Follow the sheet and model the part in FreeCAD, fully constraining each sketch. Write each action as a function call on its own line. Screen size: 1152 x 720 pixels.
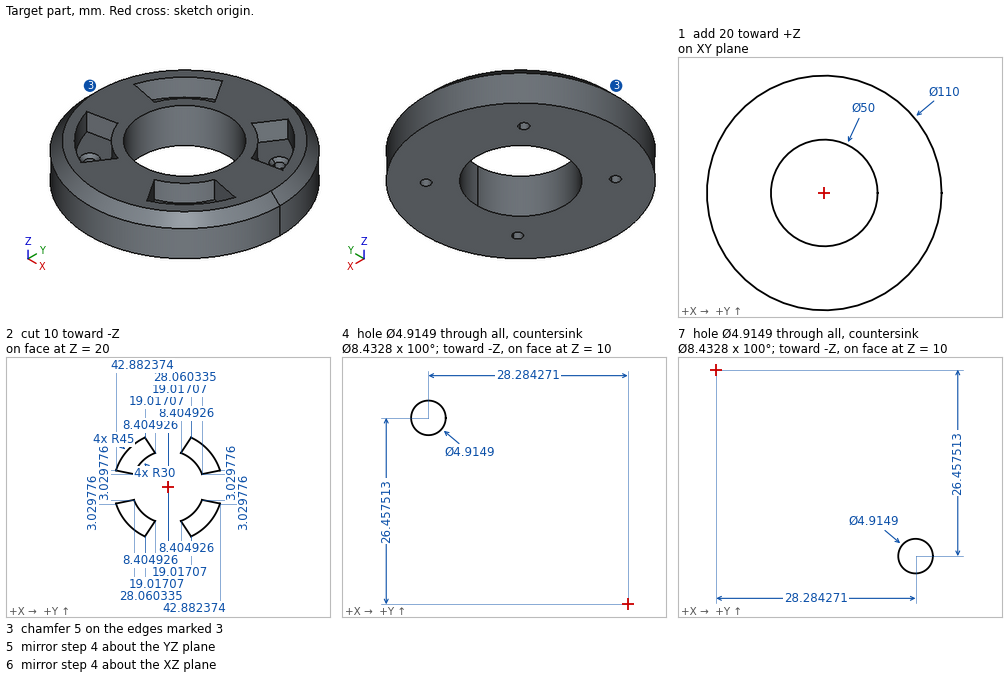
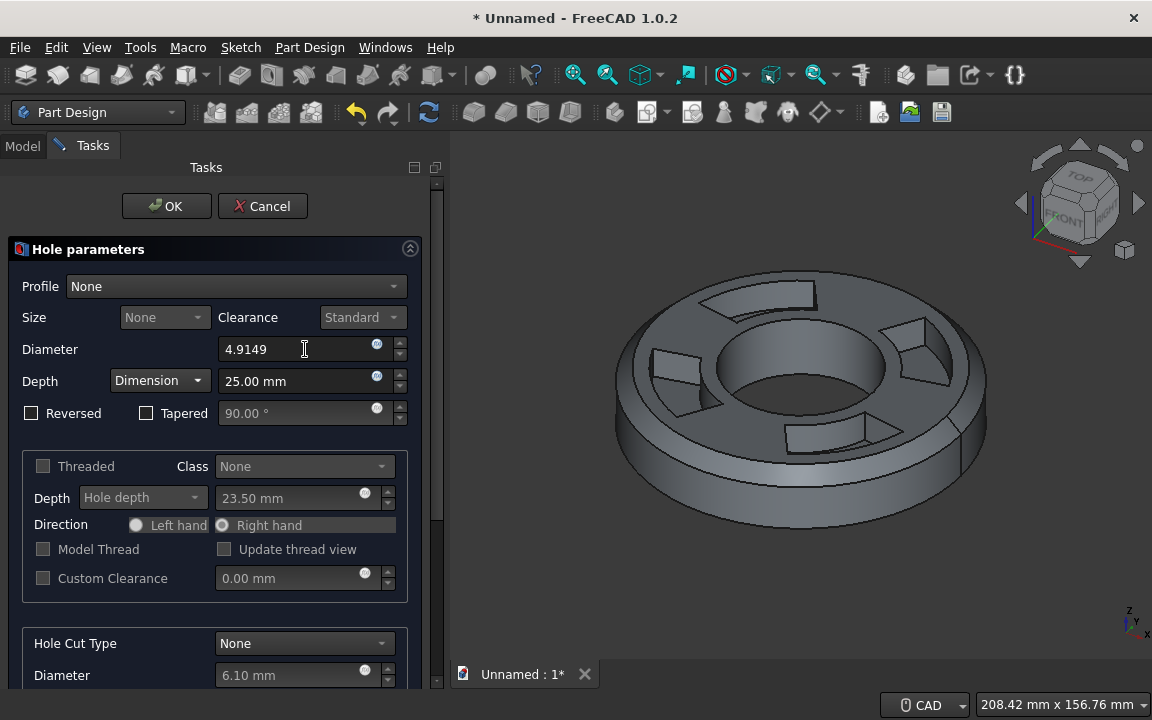
click(161, 380)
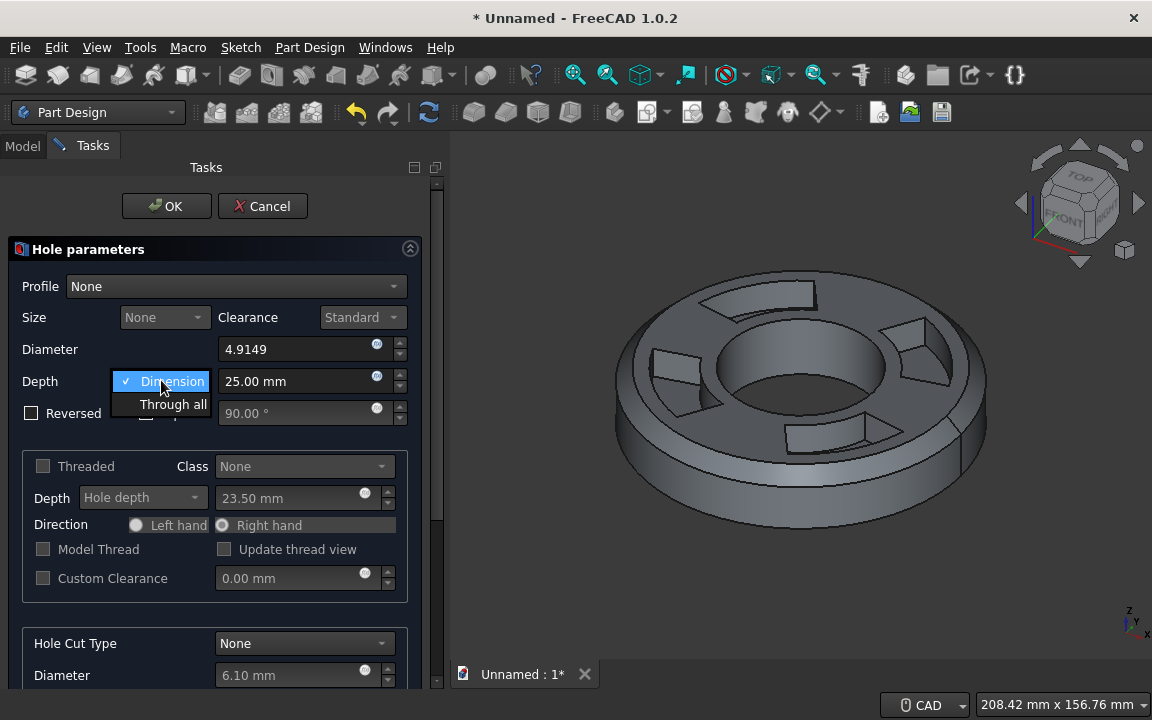
click(160, 404)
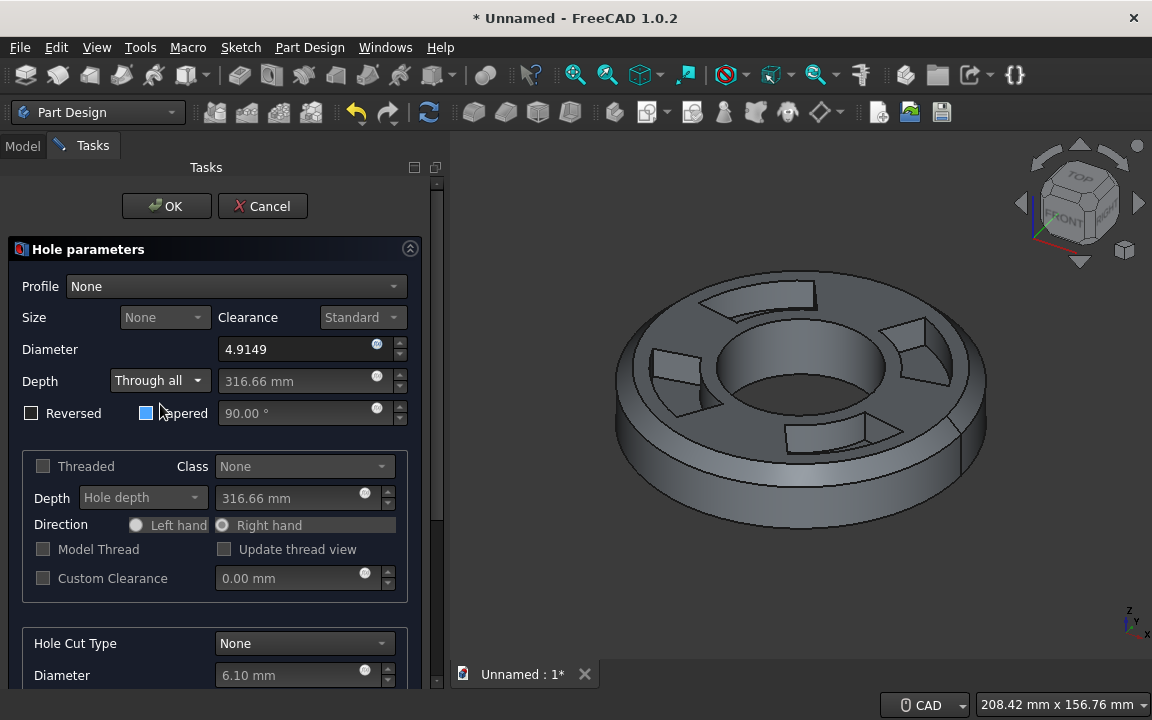
click(306, 644)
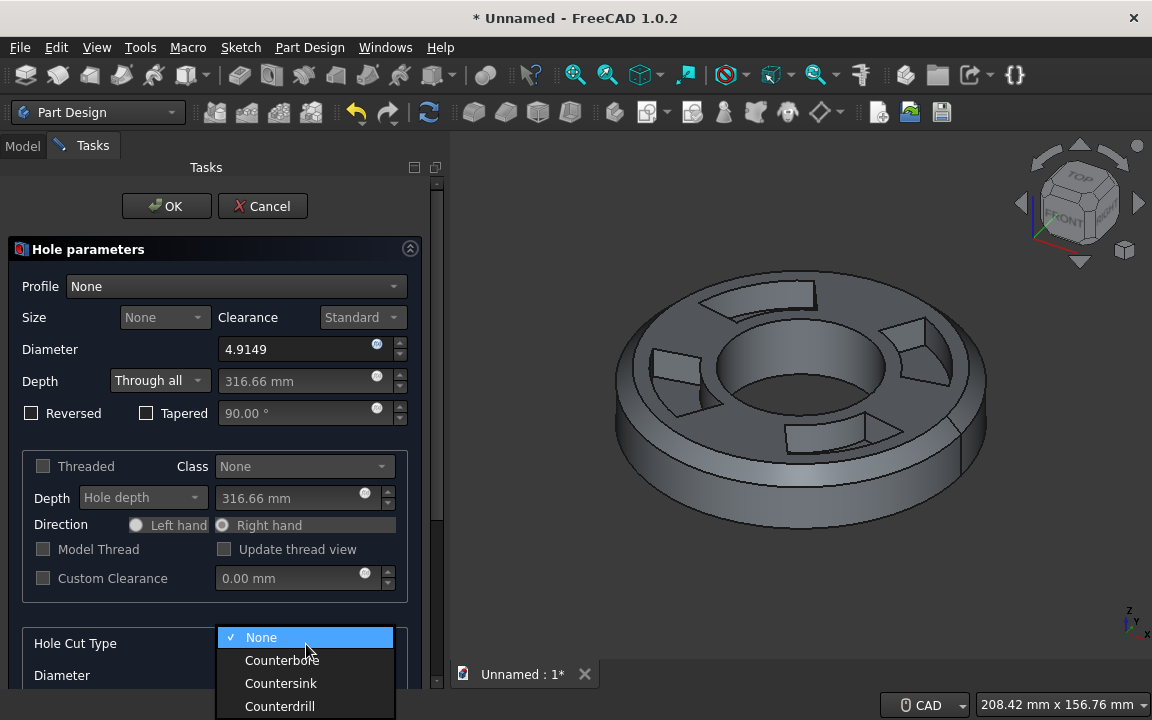
click(304, 684)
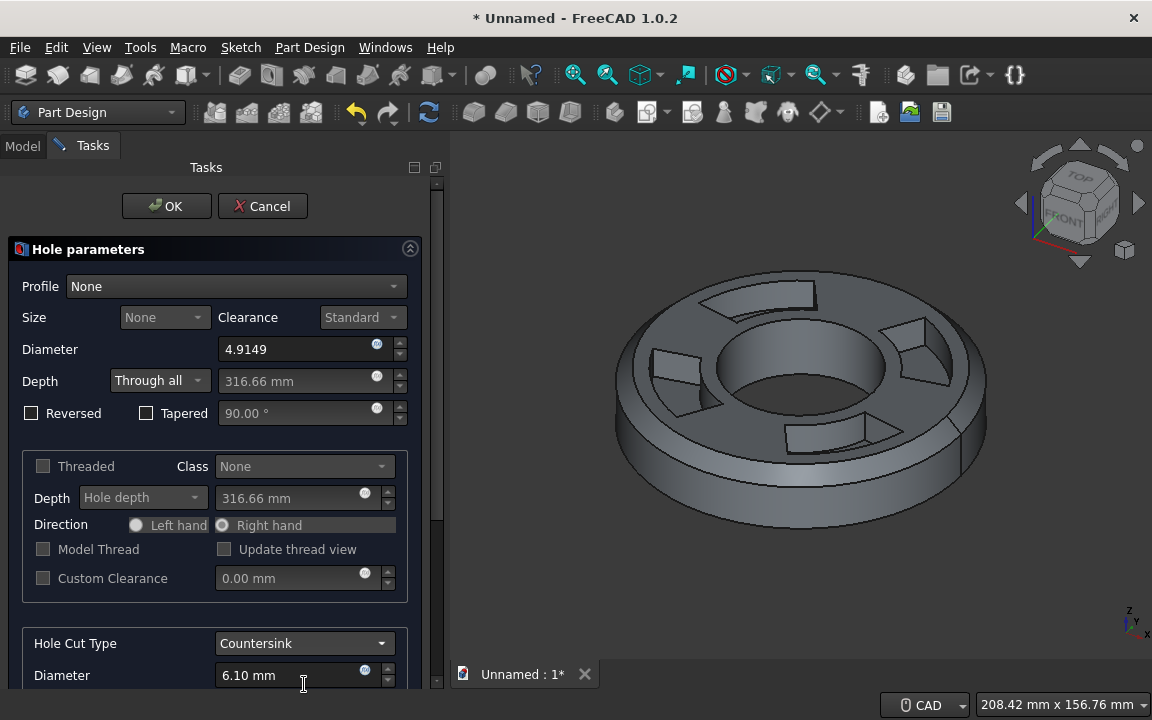
scroll(437, 432, down, 3)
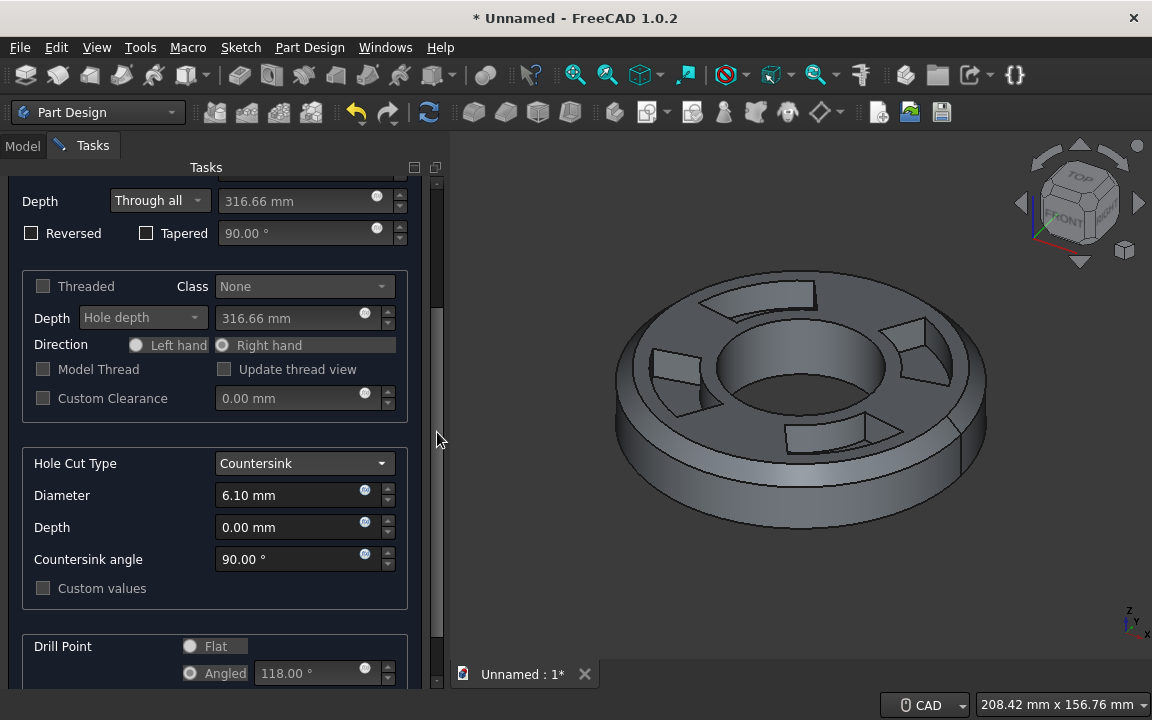
triple_click(298, 559)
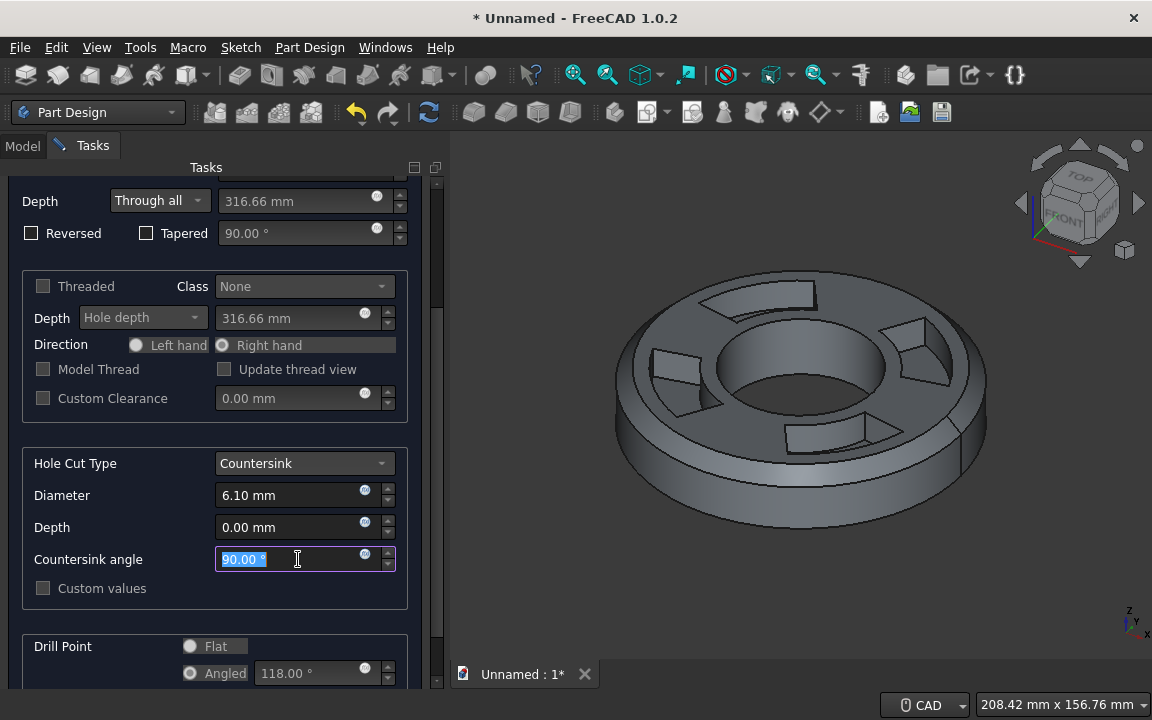
text(100)
key(Tab)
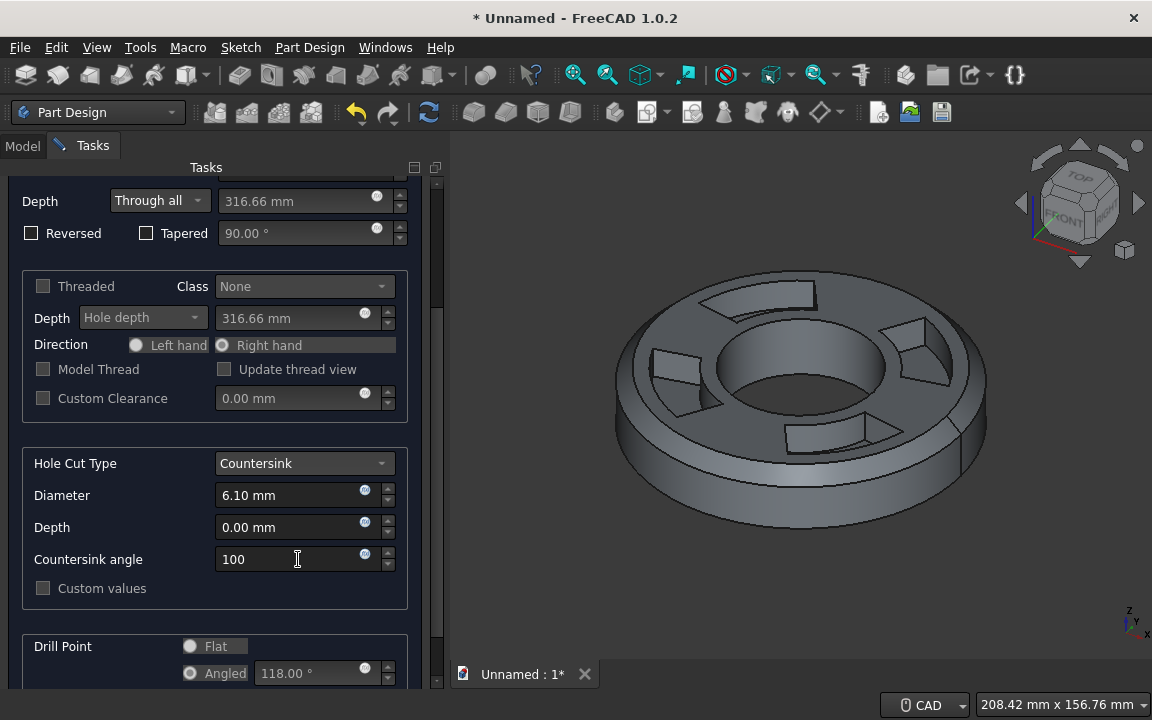
triple_click(298, 495)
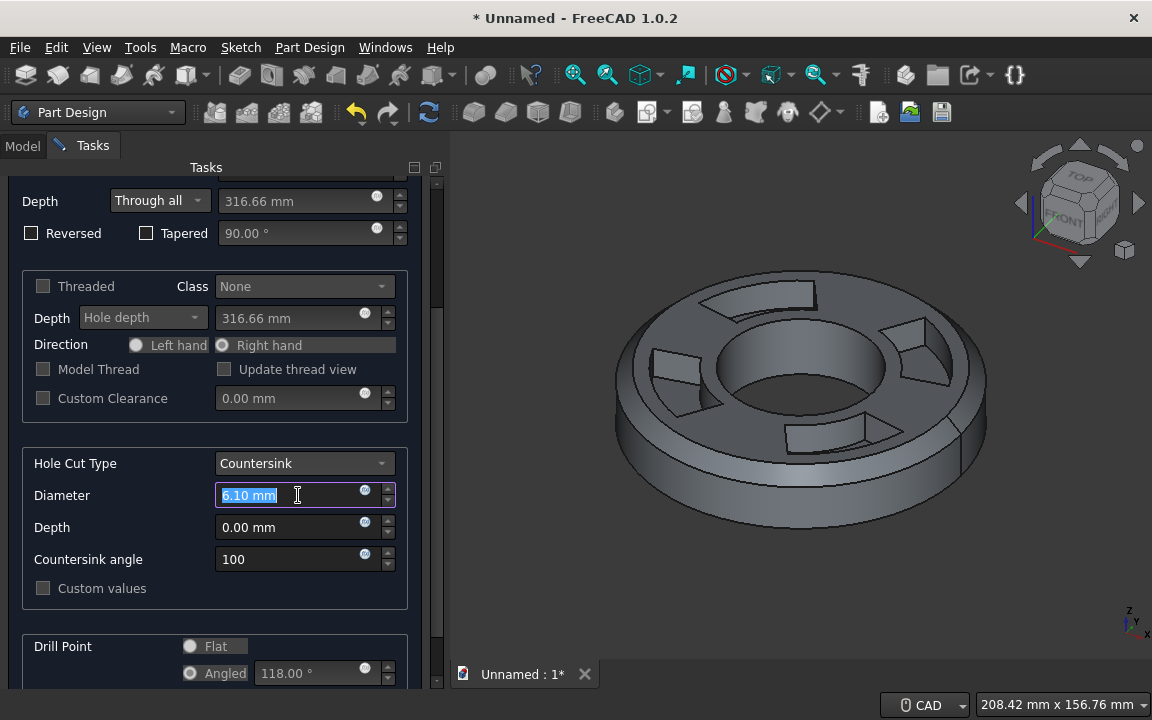
text(8.4328)
key(Tab)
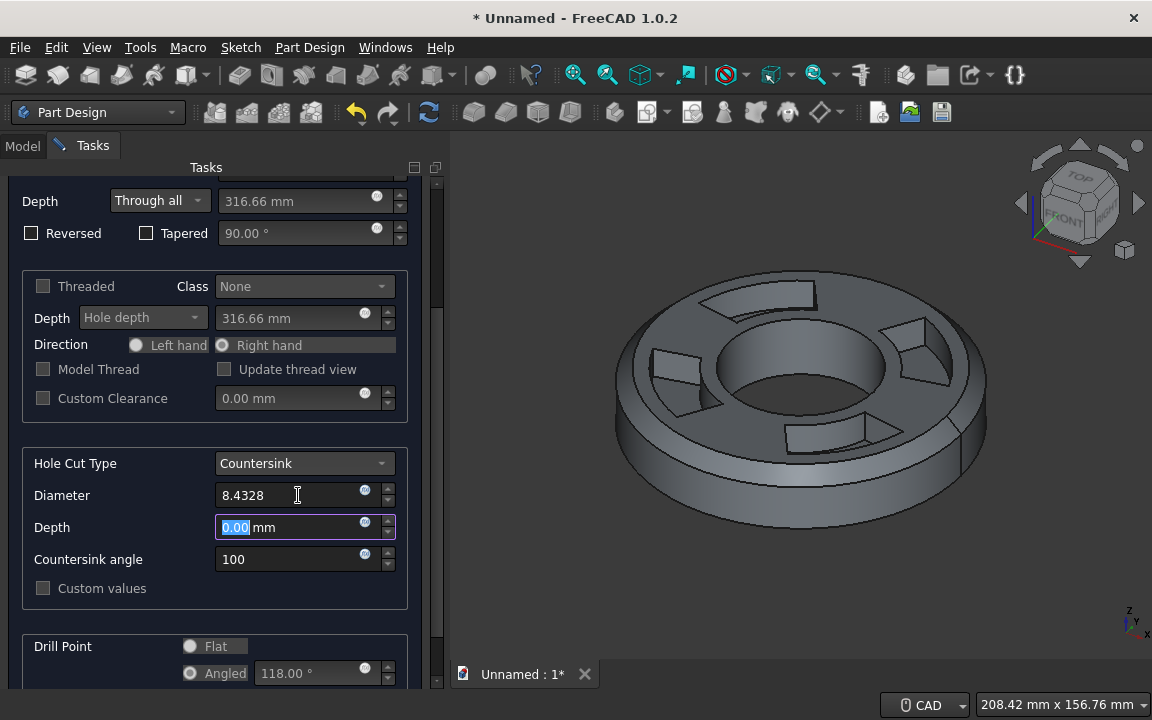
scroll(437, 432, up, 4)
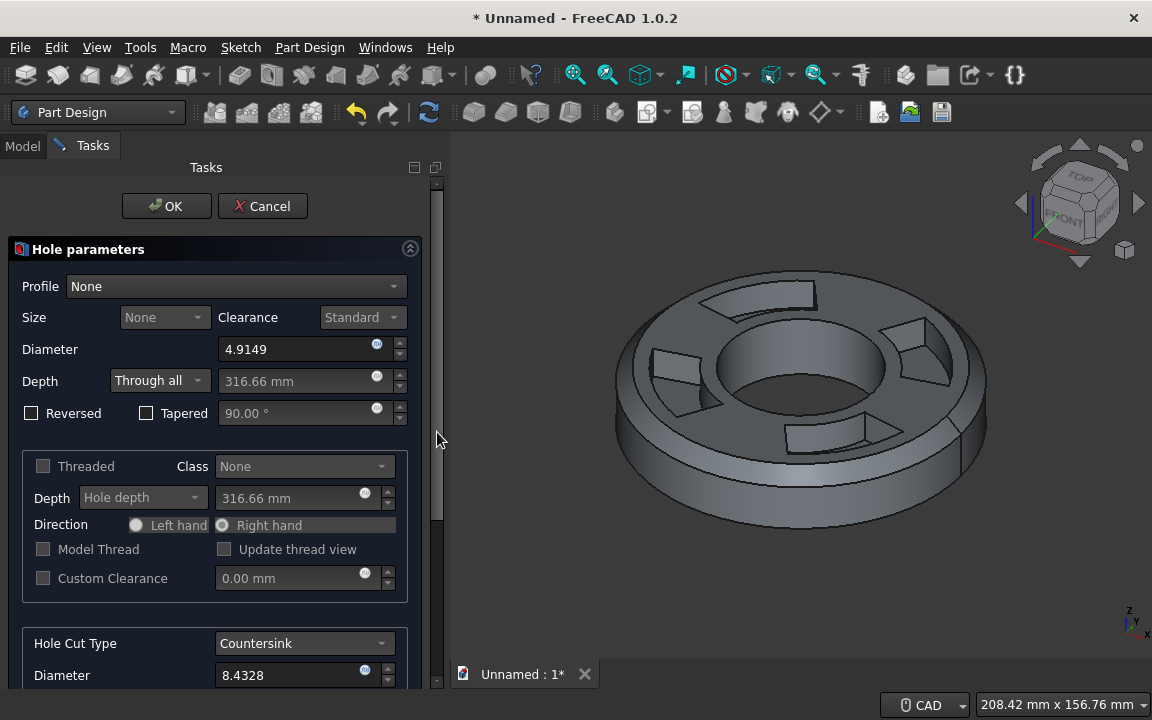
click(167, 206)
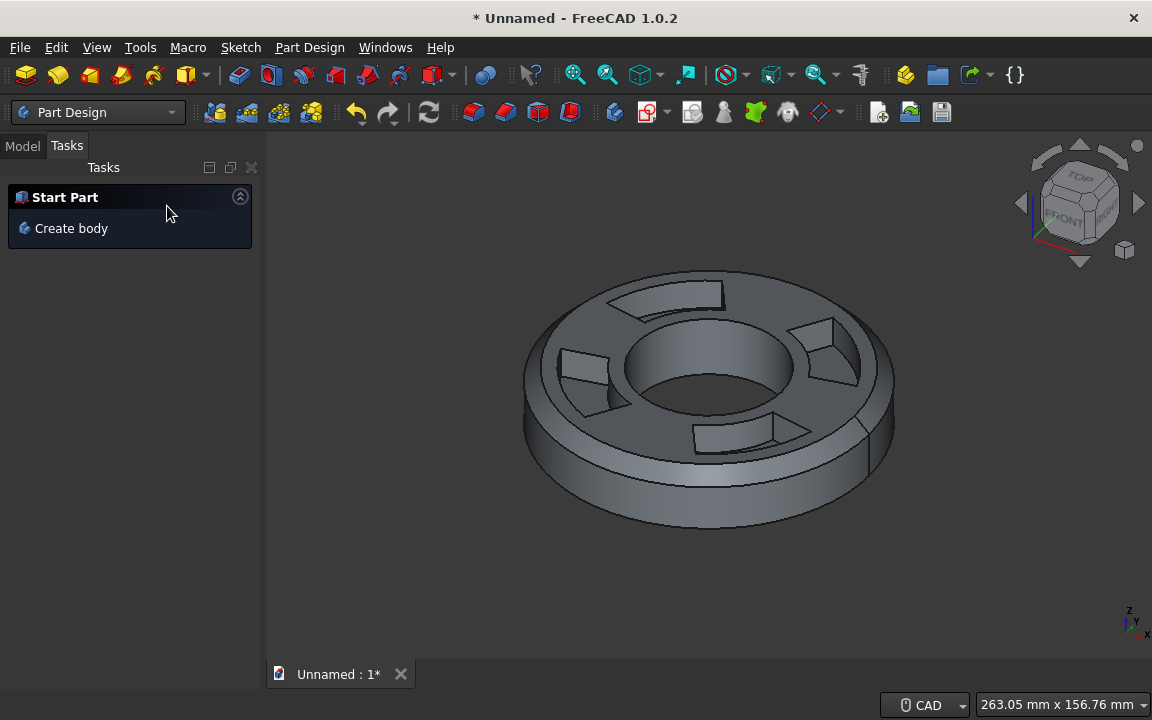
click(23, 145)